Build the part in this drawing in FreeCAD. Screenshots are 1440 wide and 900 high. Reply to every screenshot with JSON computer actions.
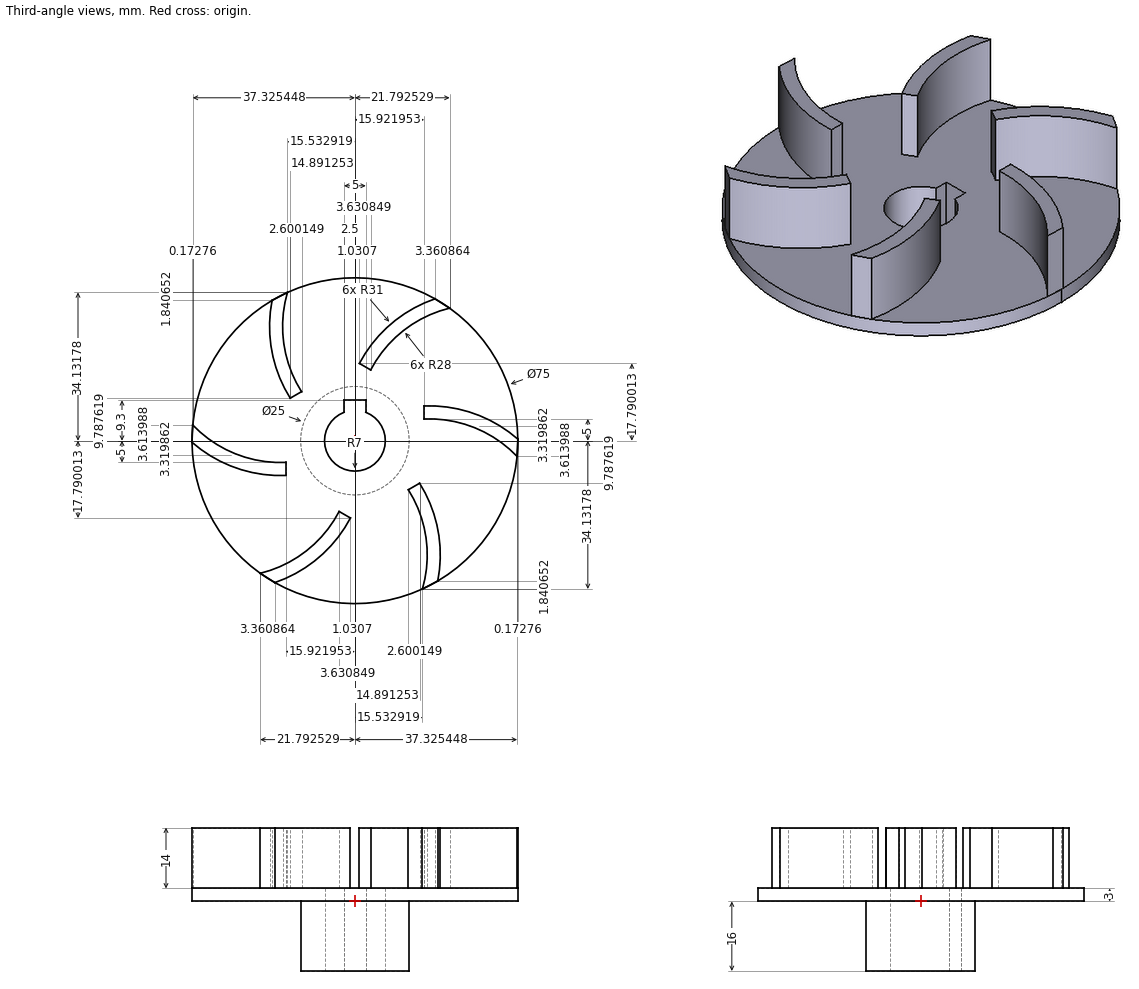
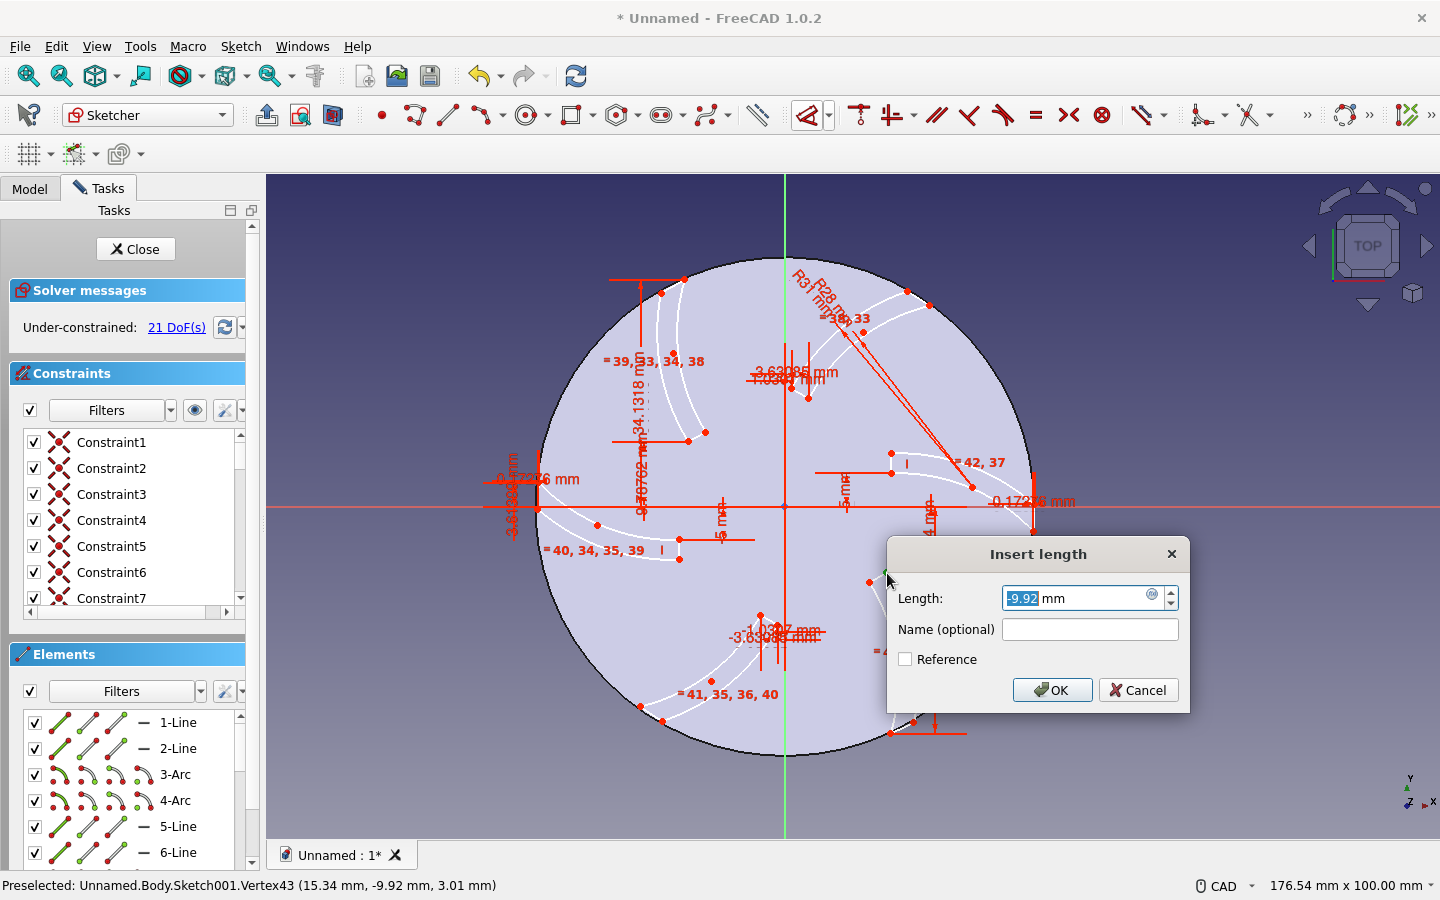
{"action": "type", "text": "-9.787619"}
{"action": "key", "text": "Return"}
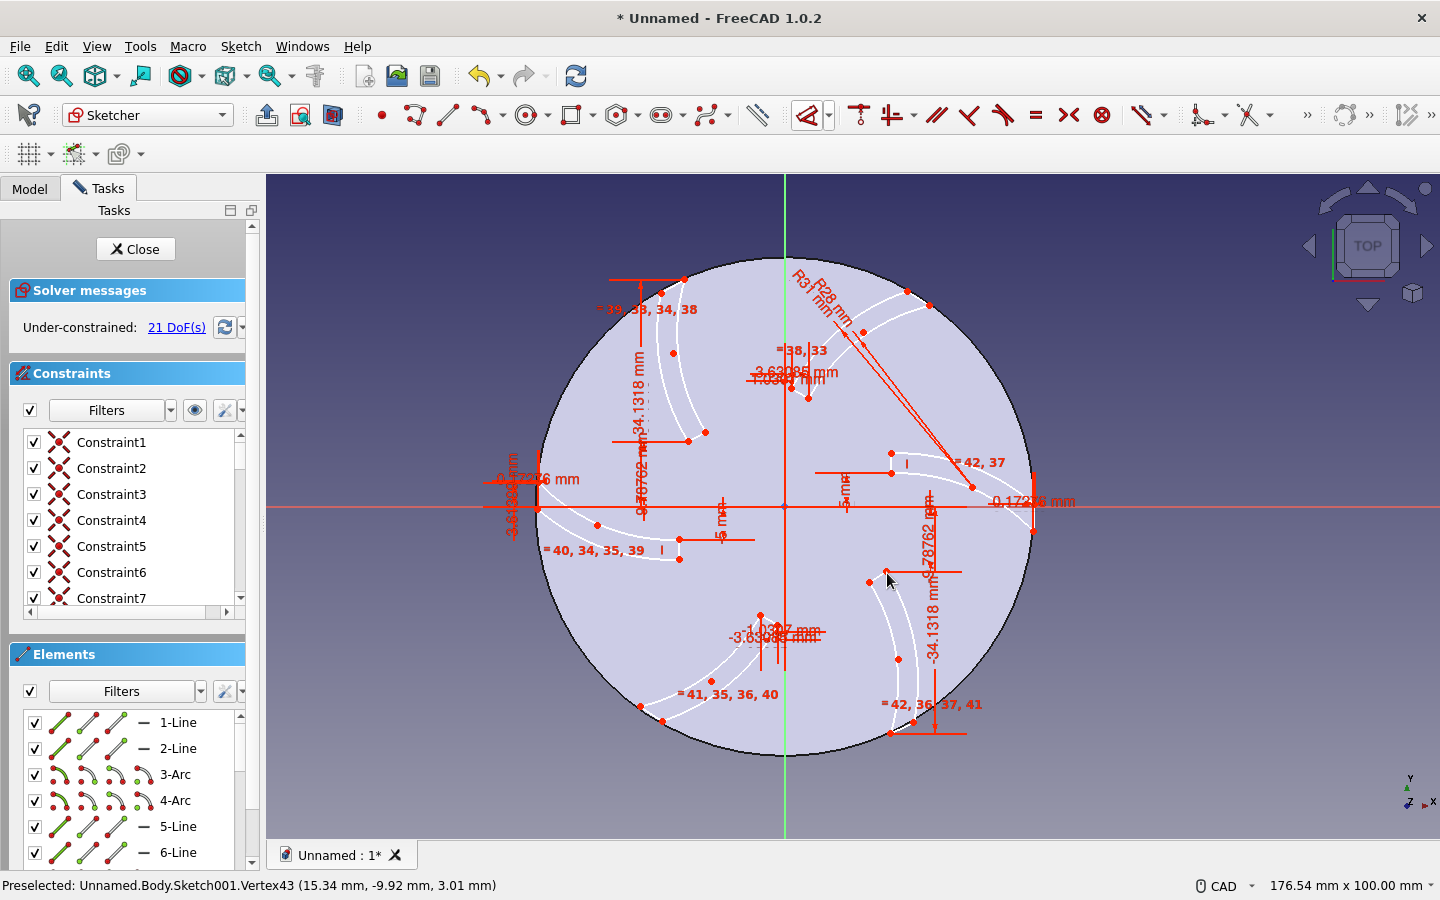
{"action": "scroll", "coordinate": [1033, 532], "scroll_direction": "up", "scroll_amount": 3}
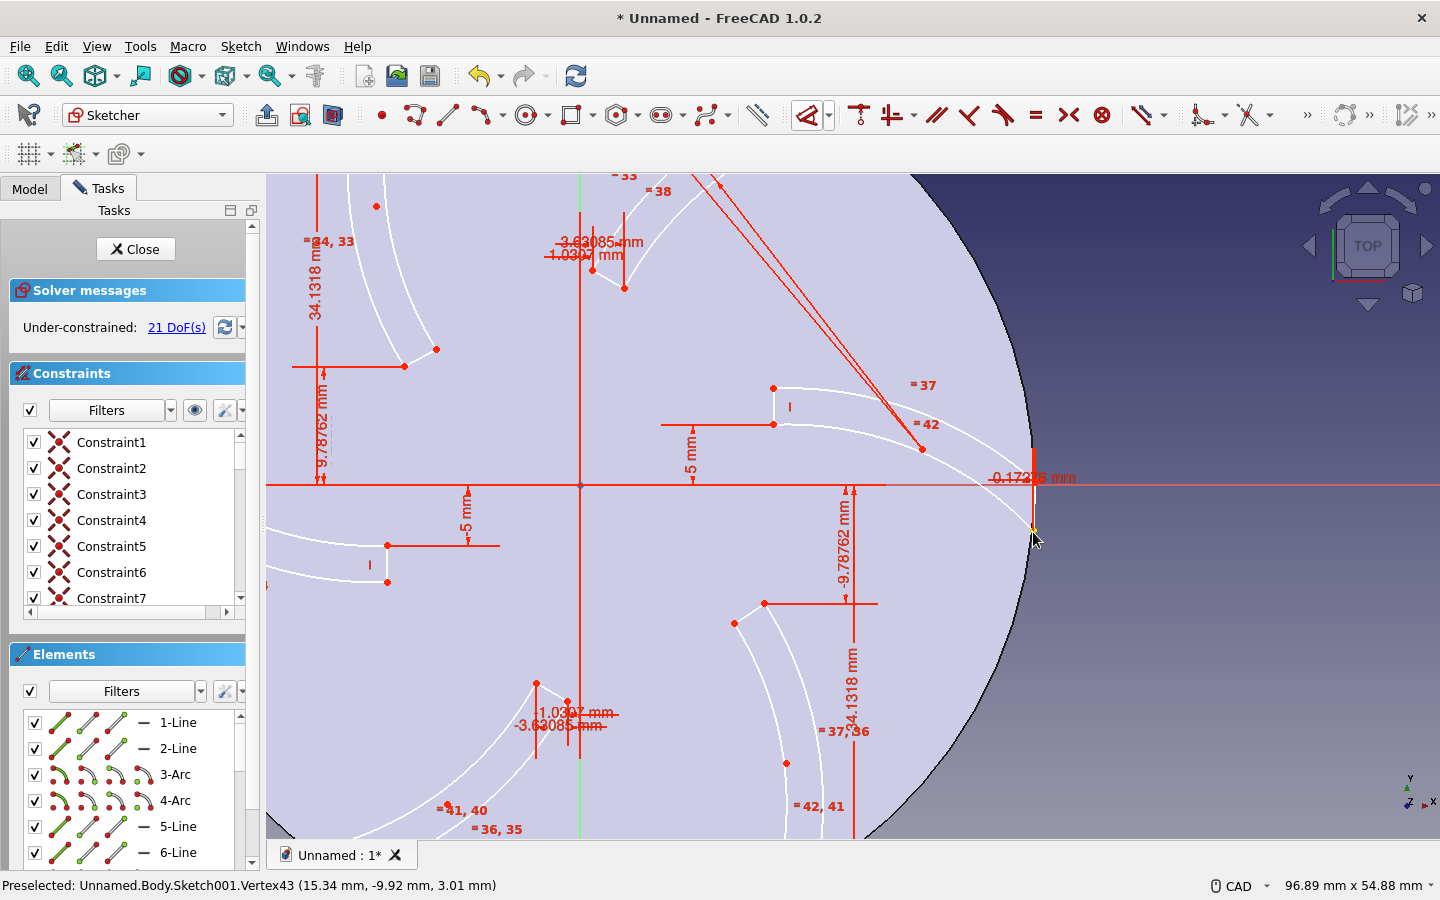
{"action": "left_click", "coordinate": [1033, 531]}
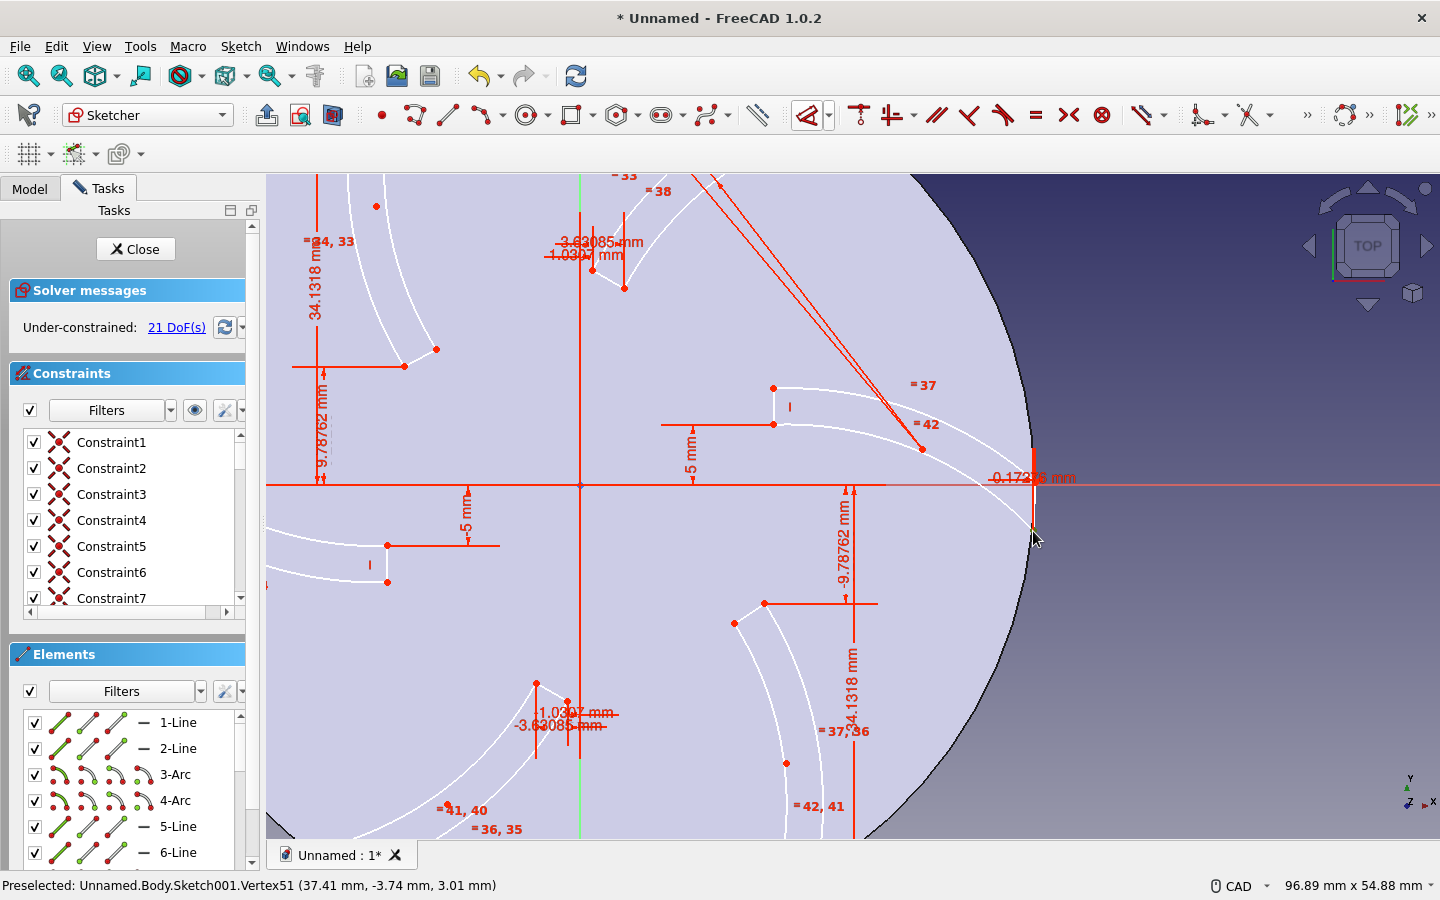
{"action": "key", "text": "i"}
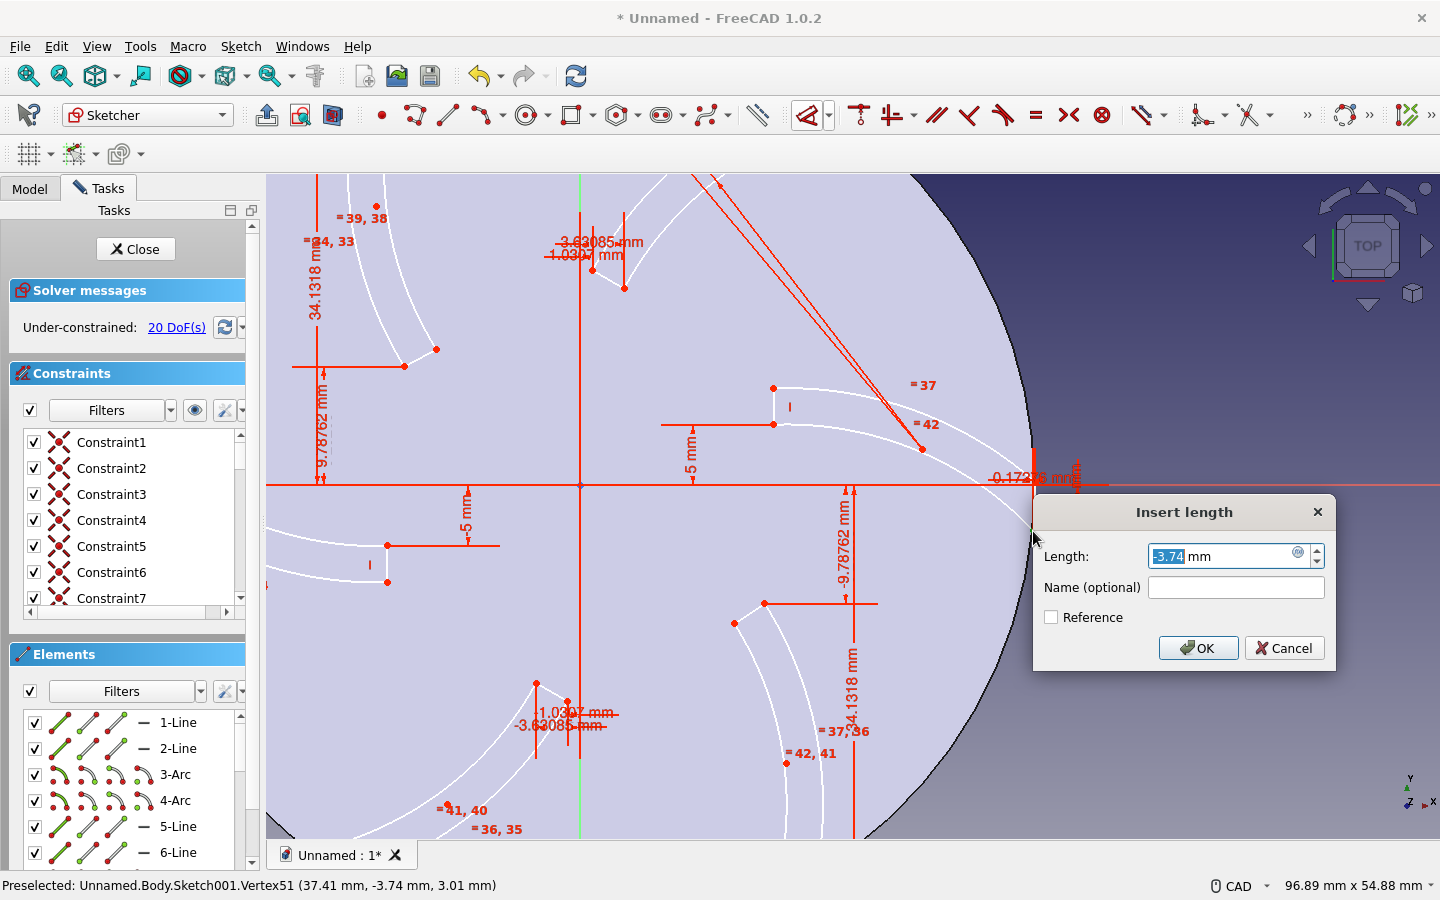
{"action": "type", "text": "-3.613988"}
{"action": "key", "text": "Return"}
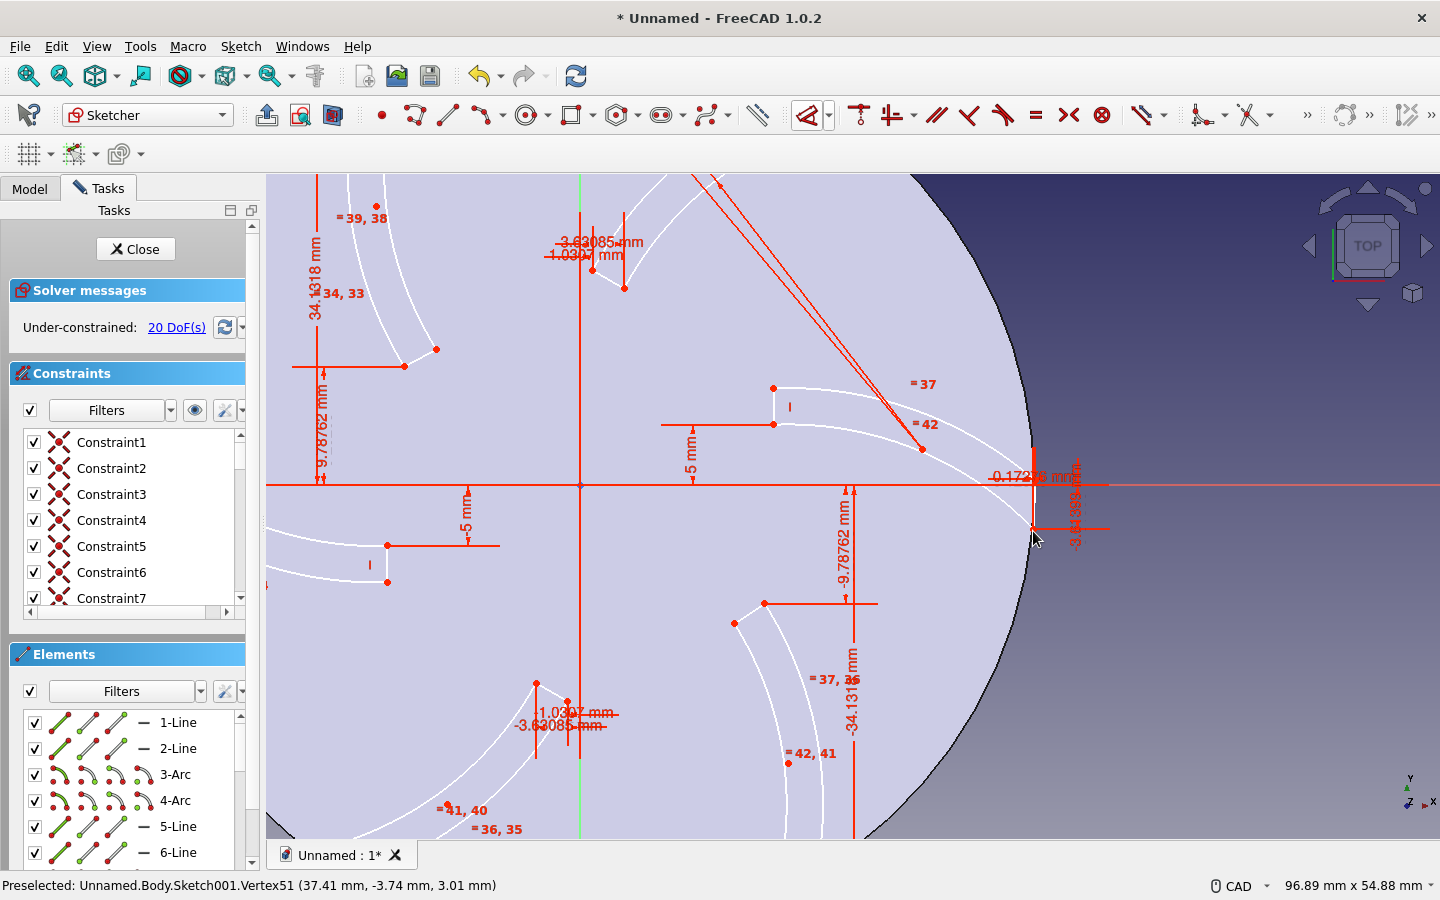
{"action": "scroll", "coordinate": [1033, 532], "scroll_direction": "down", "scroll_amount": 3}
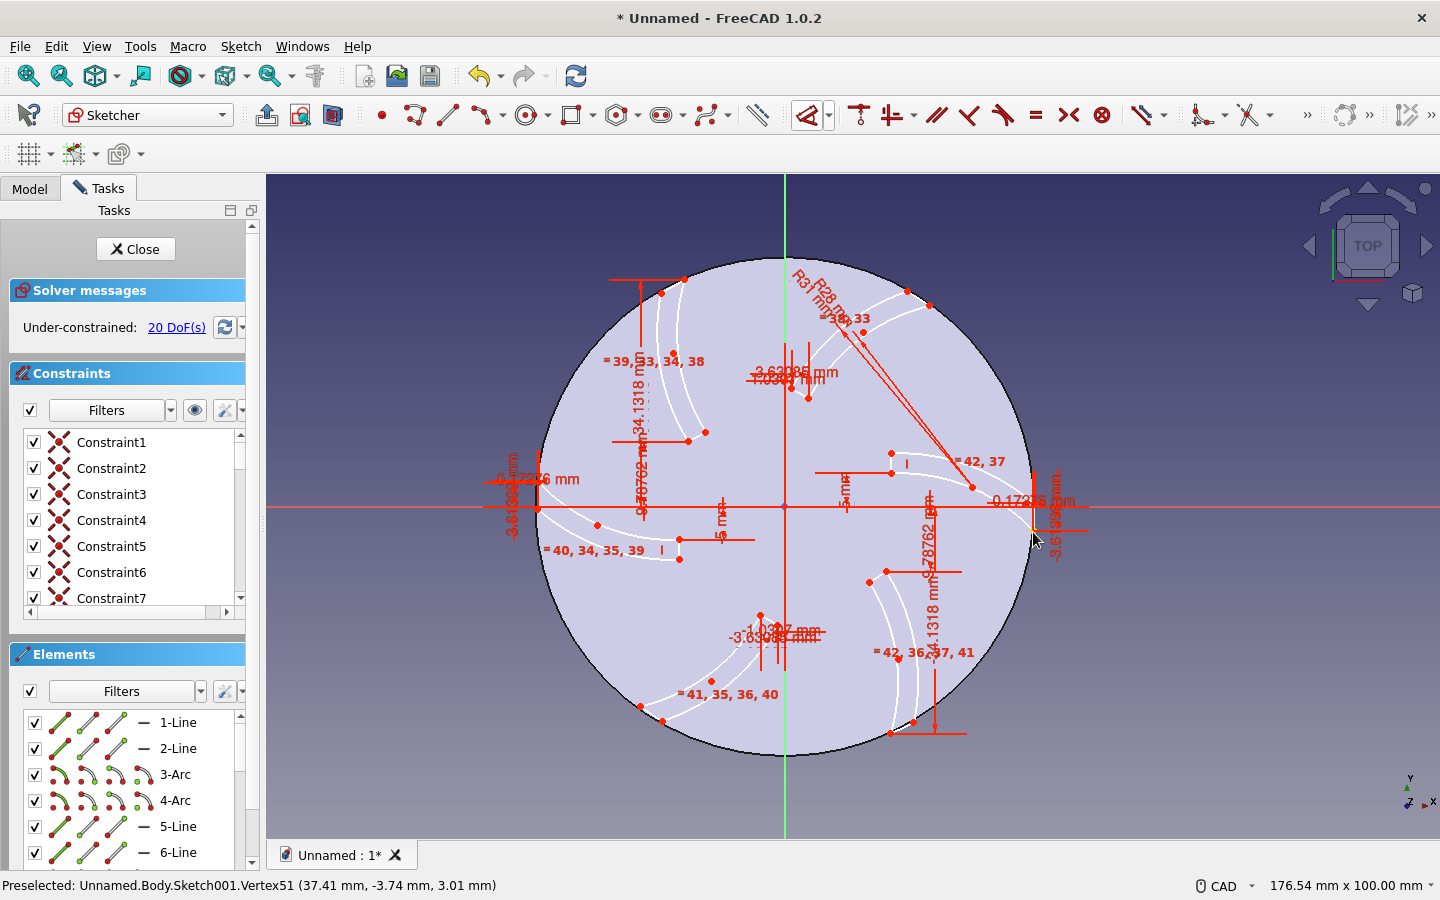
{"action": "scroll", "coordinate": [923, 302], "scroll_direction": "up", "scroll_amount": 5}